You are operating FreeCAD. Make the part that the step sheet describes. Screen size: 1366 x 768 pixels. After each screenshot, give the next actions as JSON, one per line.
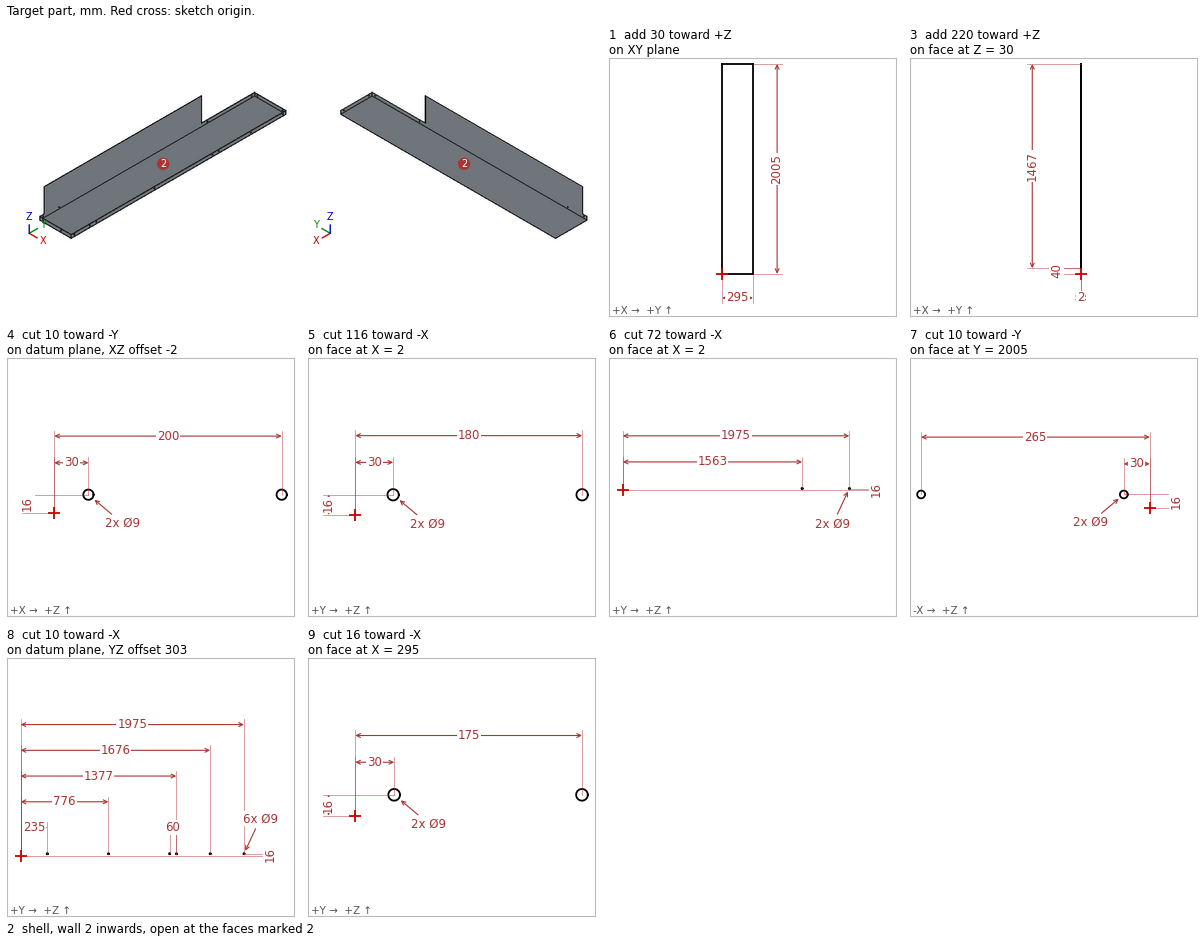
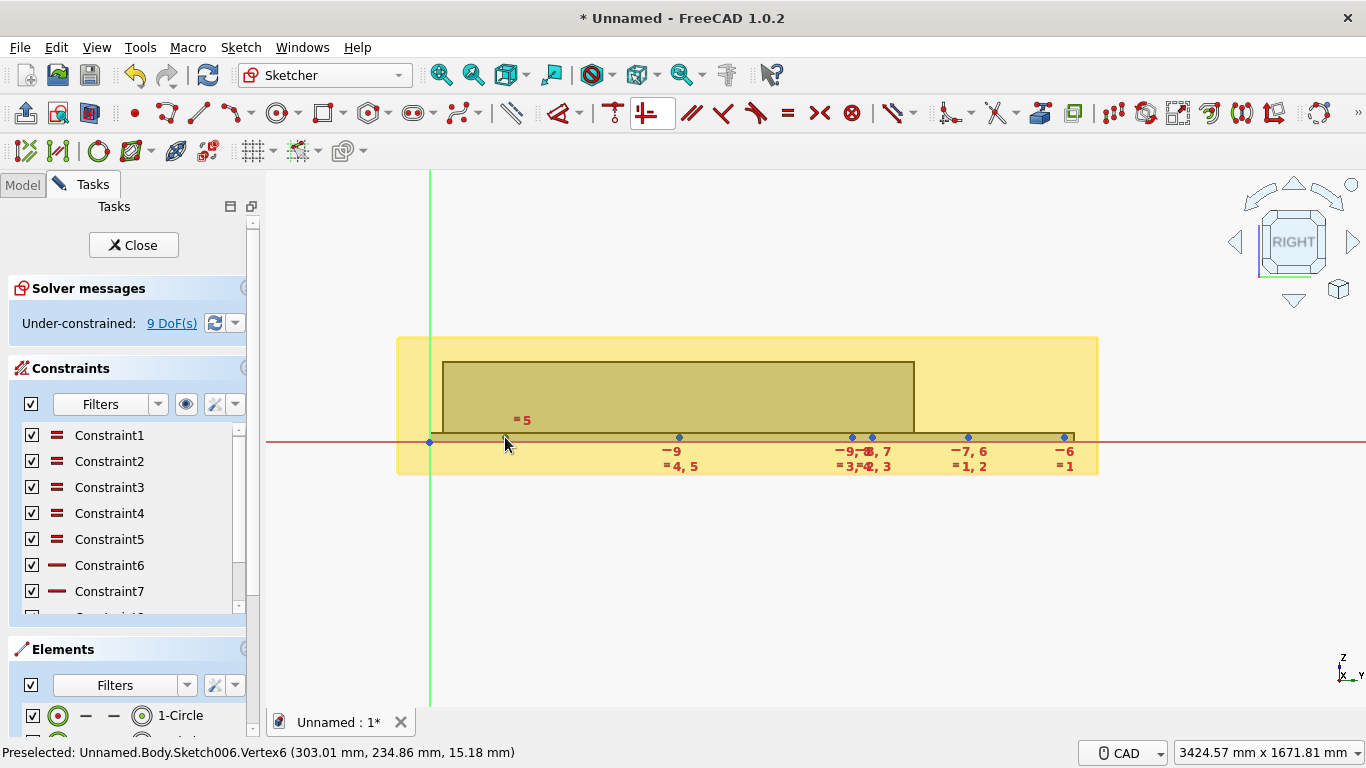
{"action": "key", "text": "h"}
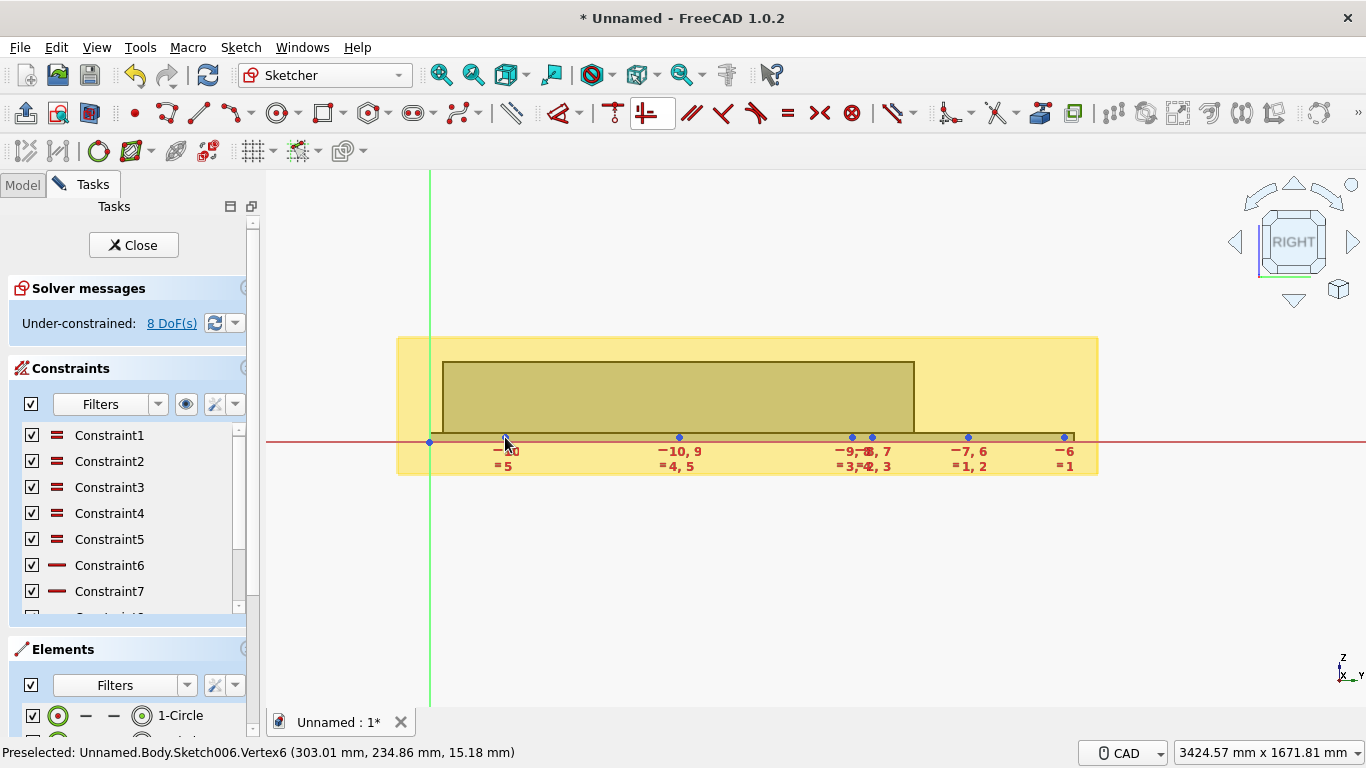
{"action": "left_click", "coordinate": [558, 114]}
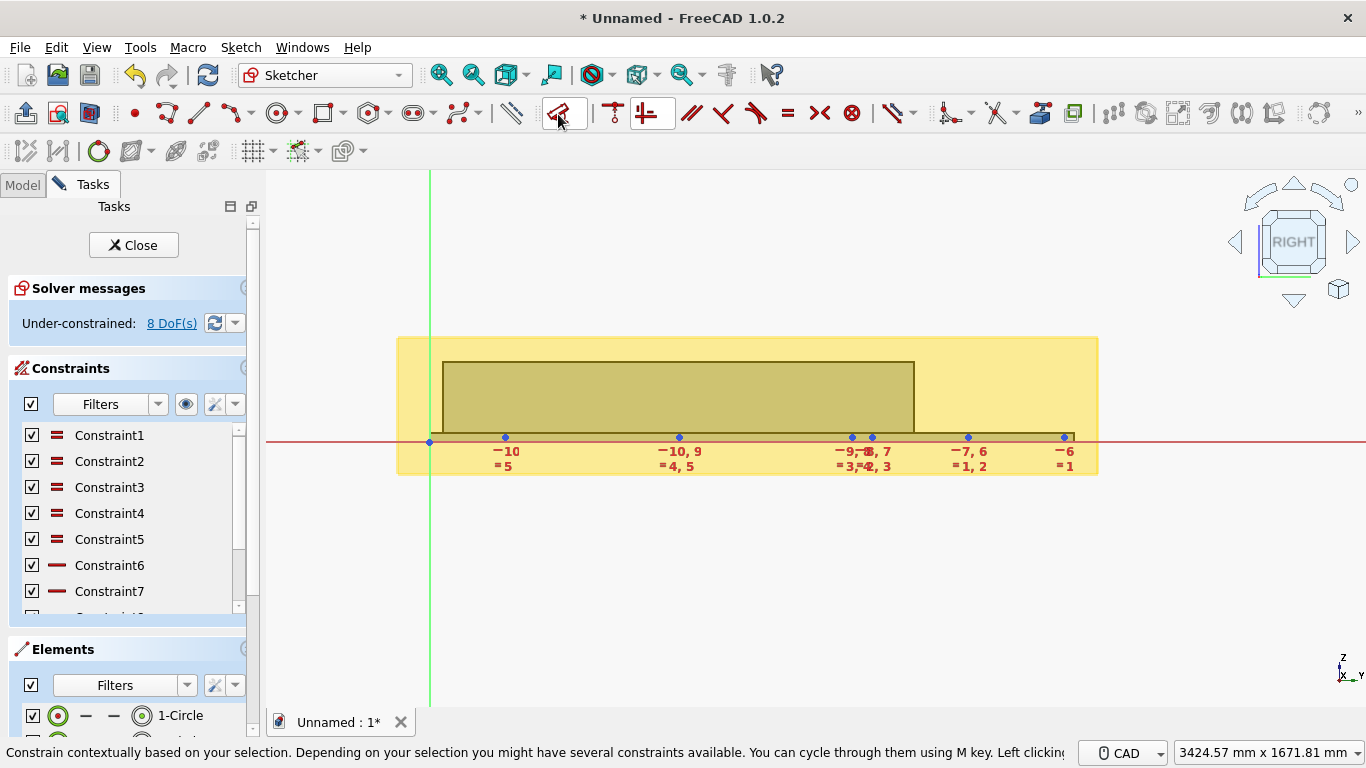
{"action": "scroll", "coordinate": [1065, 439], "scroll_direction": "up", "scroll_amount": 14}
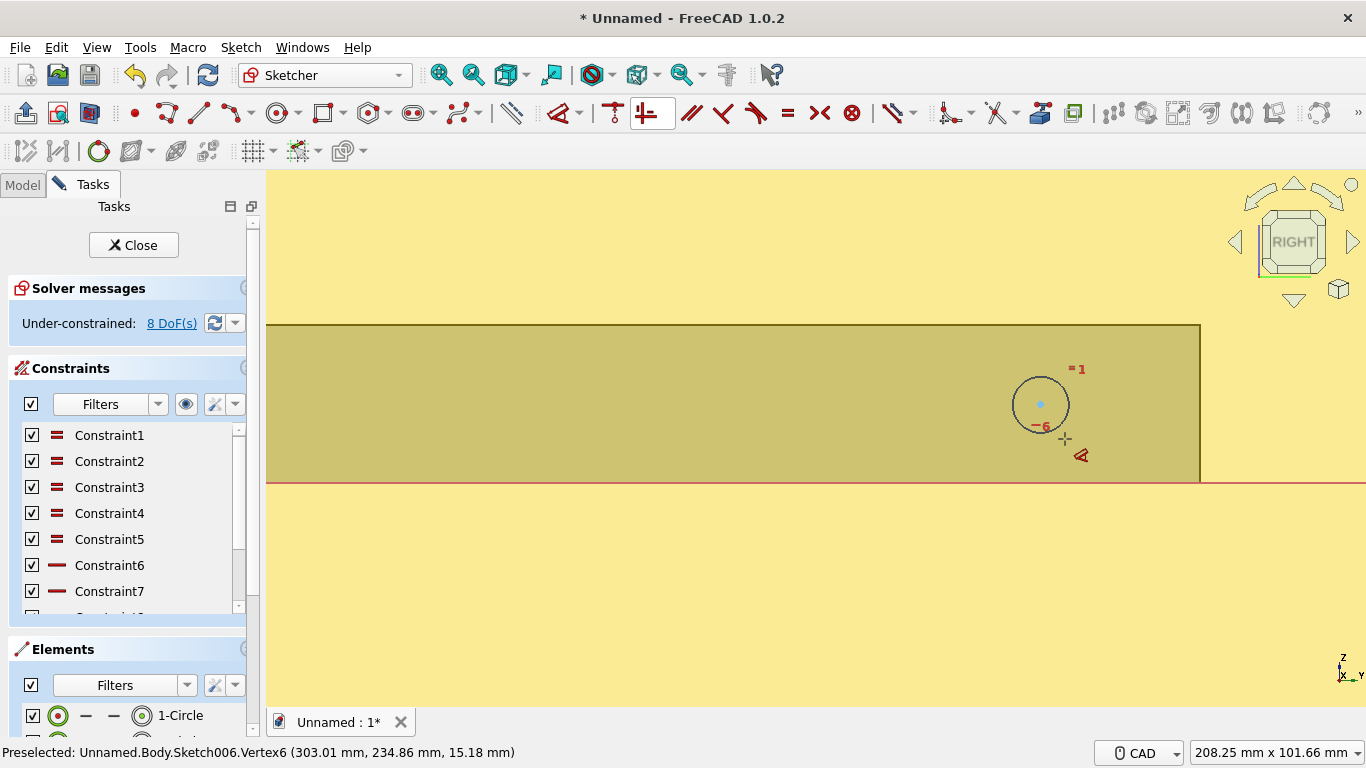
{"action": "left_click", "coordinate": [1061, 425]}
{"action": "left_click", "coordinate": [1084, 448]}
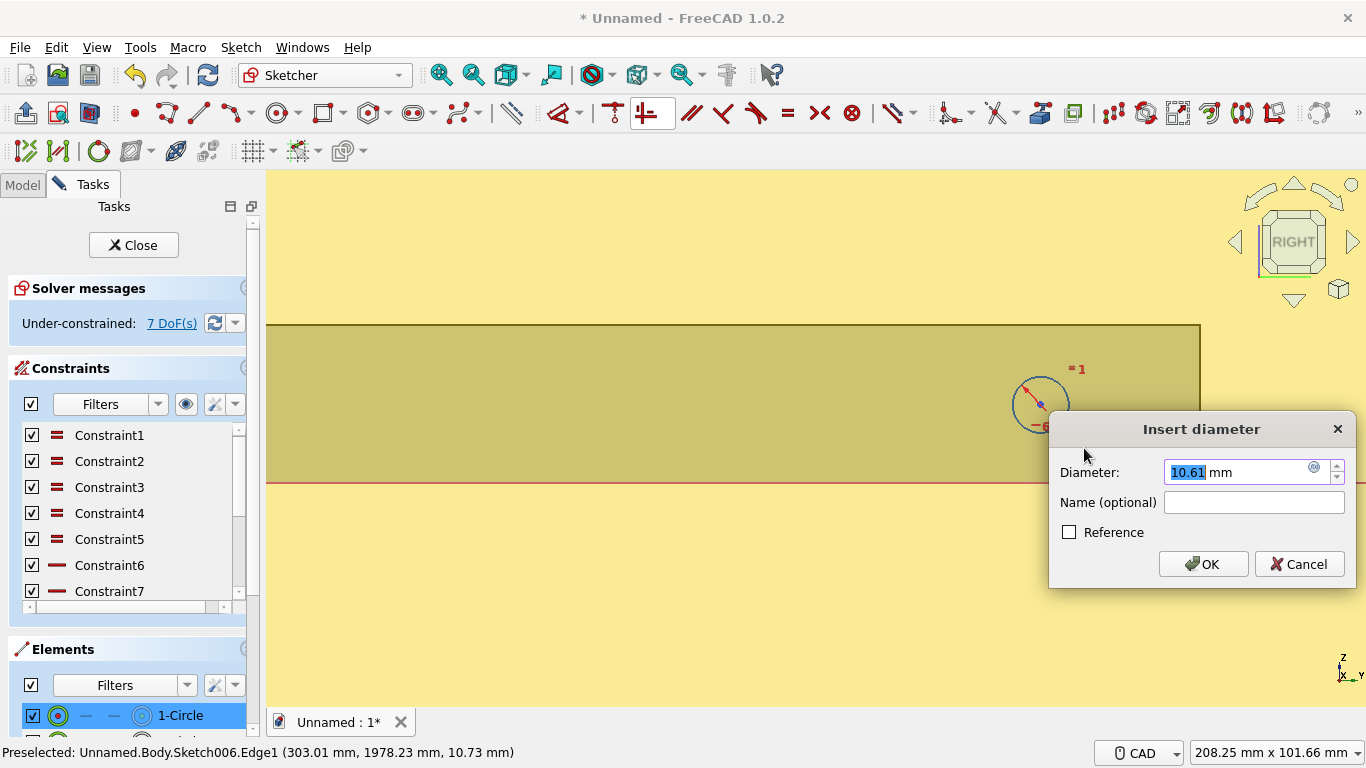
{"action": "type", "text": "9"}
{"action": "key", "text": "Return"}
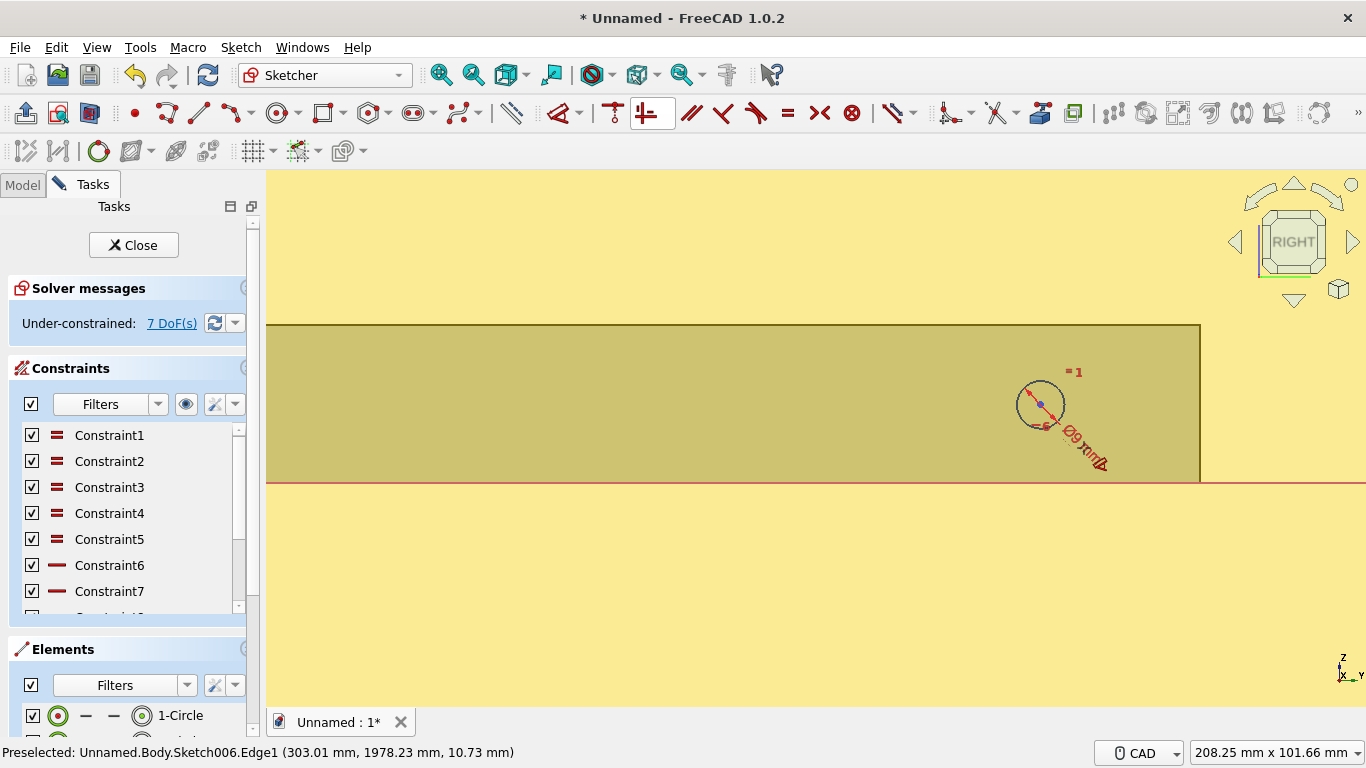
{"action": "left_click", "coordinate": [1041, 405]}
{"action": "left_click", "coordinate": [1075, 426]}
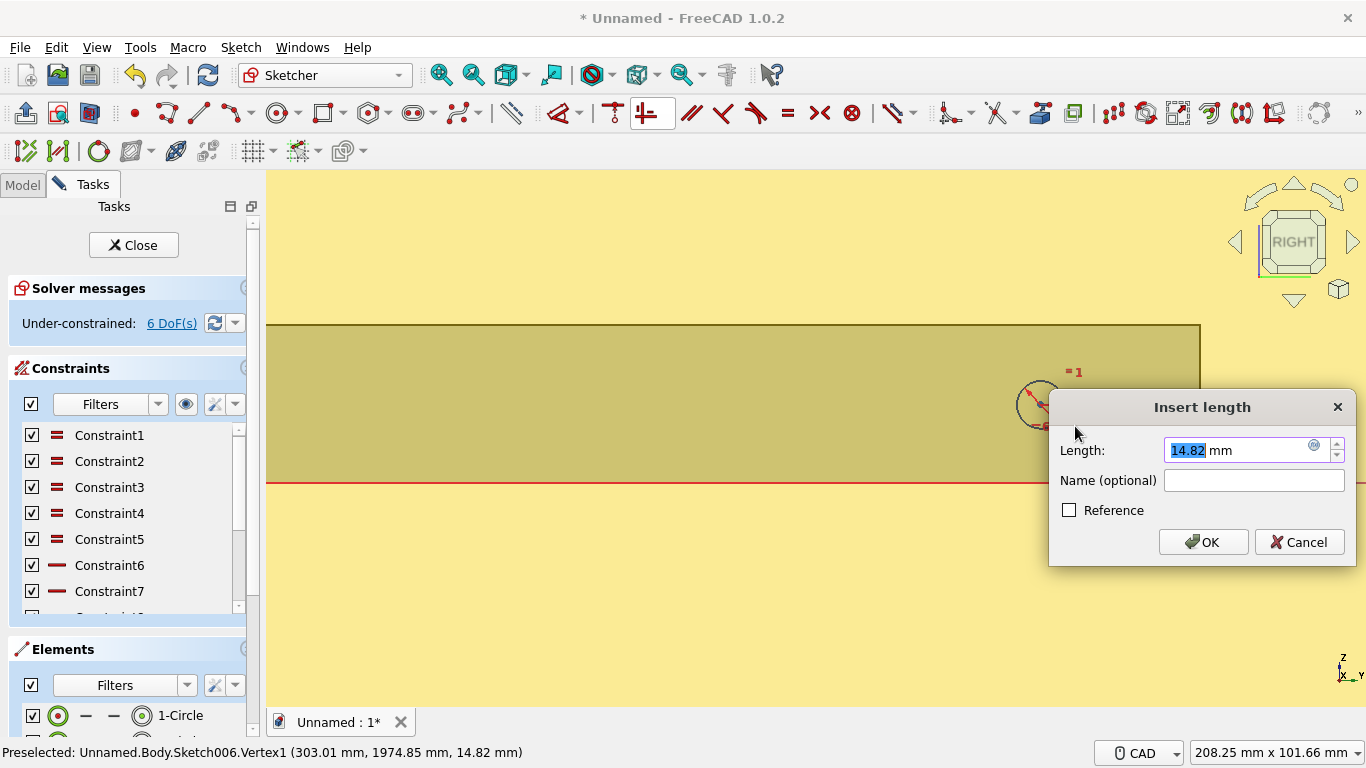
{"action": "type", "text": "16"}
{"action": "key", "text": "Return"}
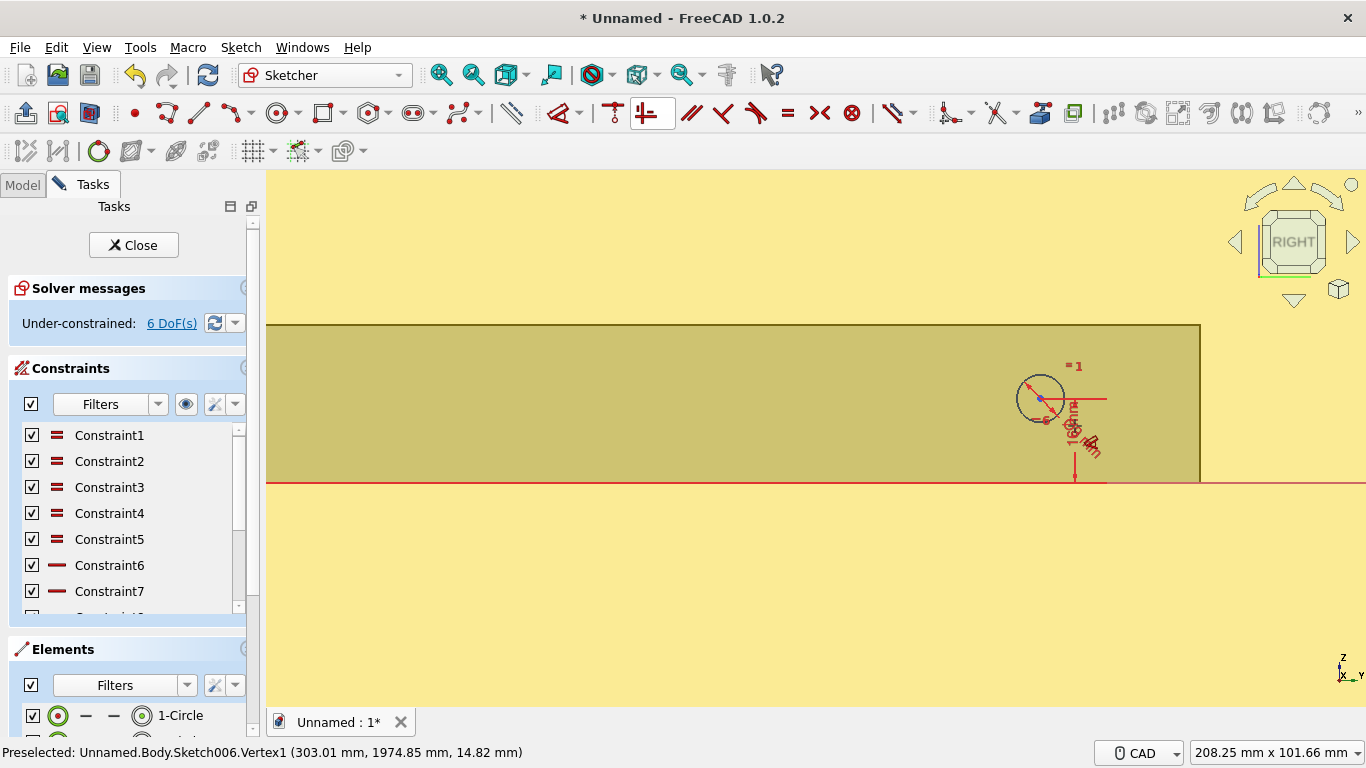
{"action": "scroll", "coordinate": [1065, 439], "scroll_direction": "down", "scroll_amount": 14}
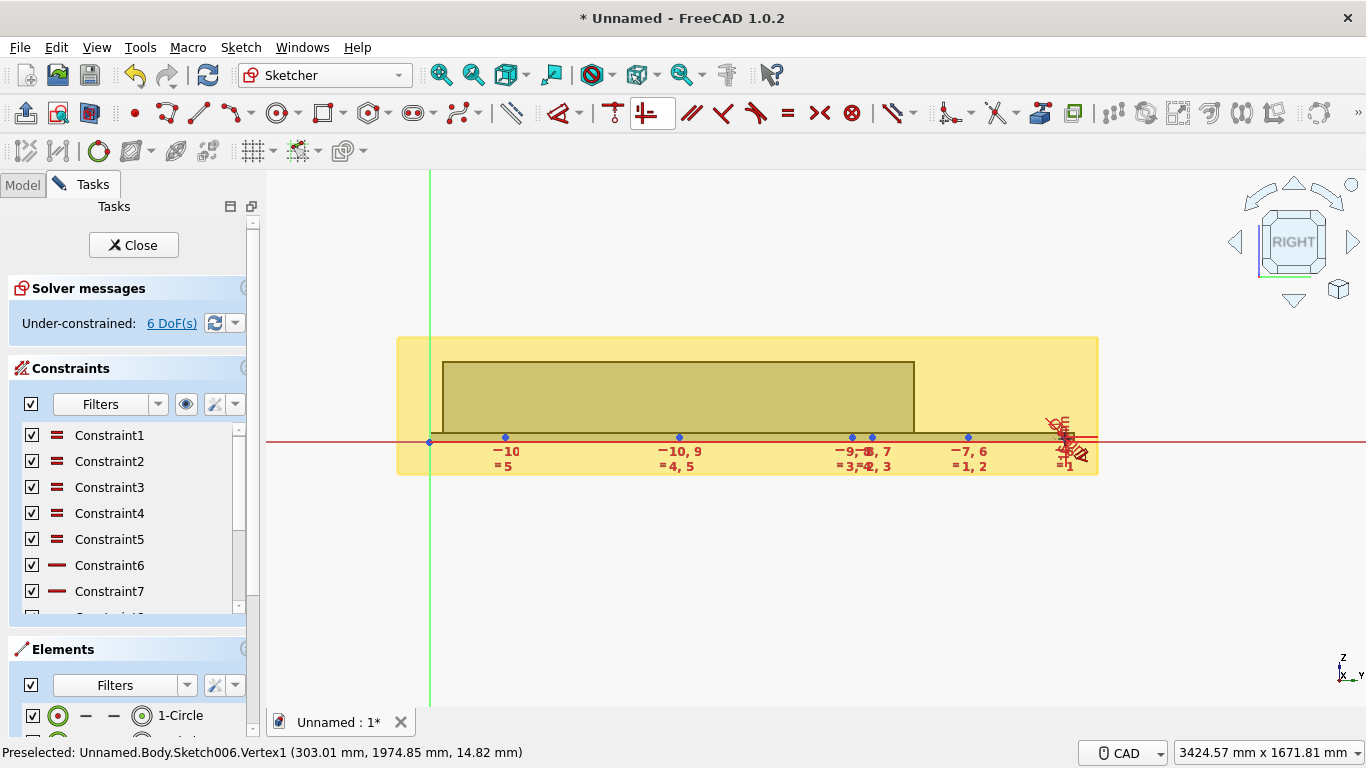
{"action": "left_click", "coordinate": [679, 437]}
{"action": "left_click", "coordinate": [554, 476]}